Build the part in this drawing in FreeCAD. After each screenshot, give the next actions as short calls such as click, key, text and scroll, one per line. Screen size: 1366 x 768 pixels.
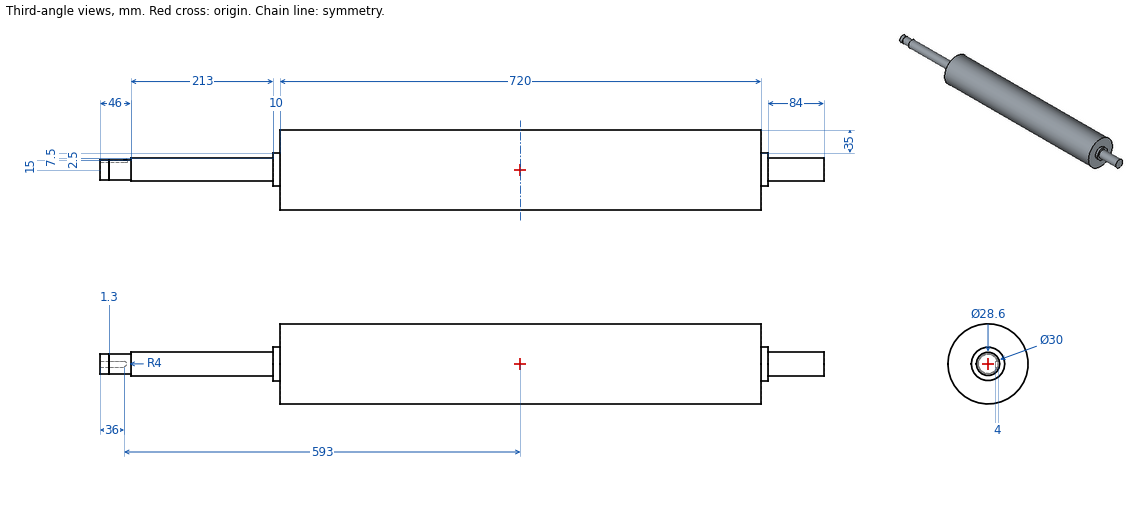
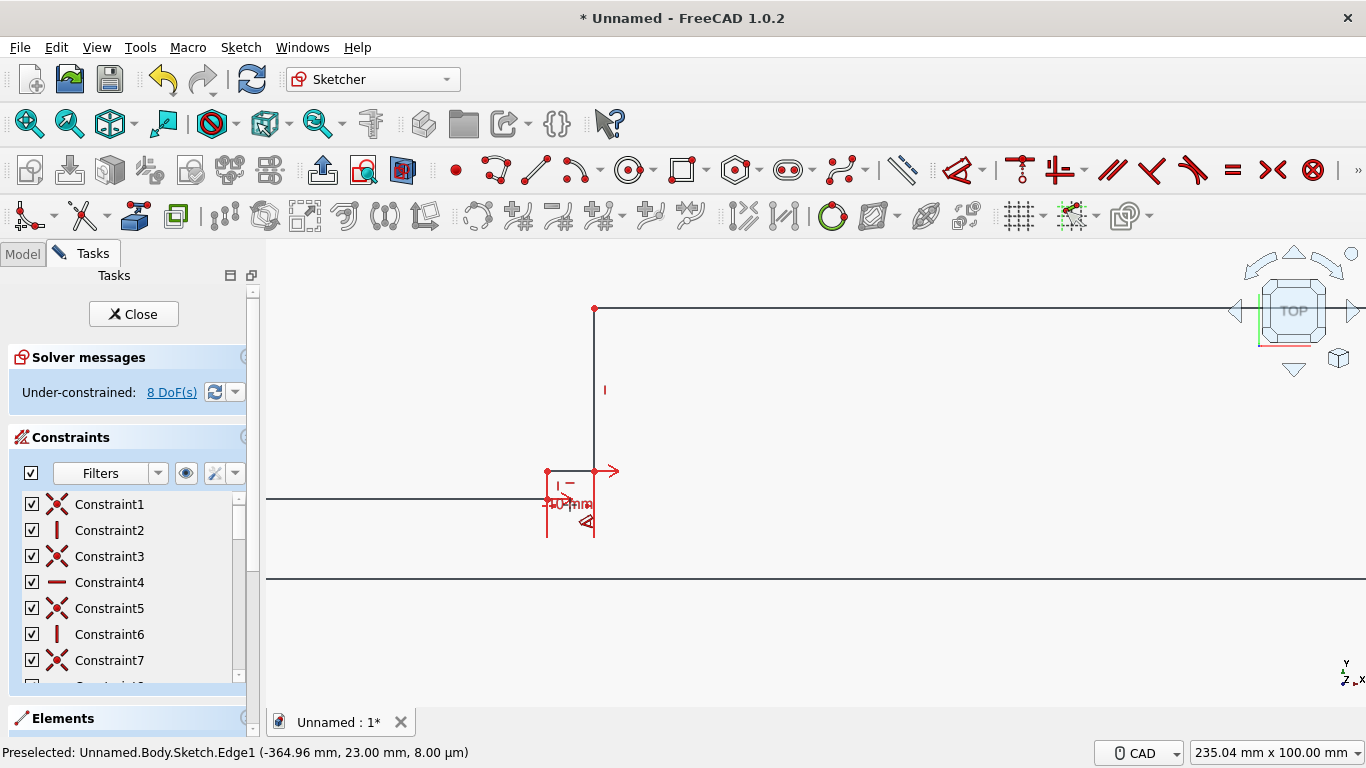
scroll(572, 478, down, 10)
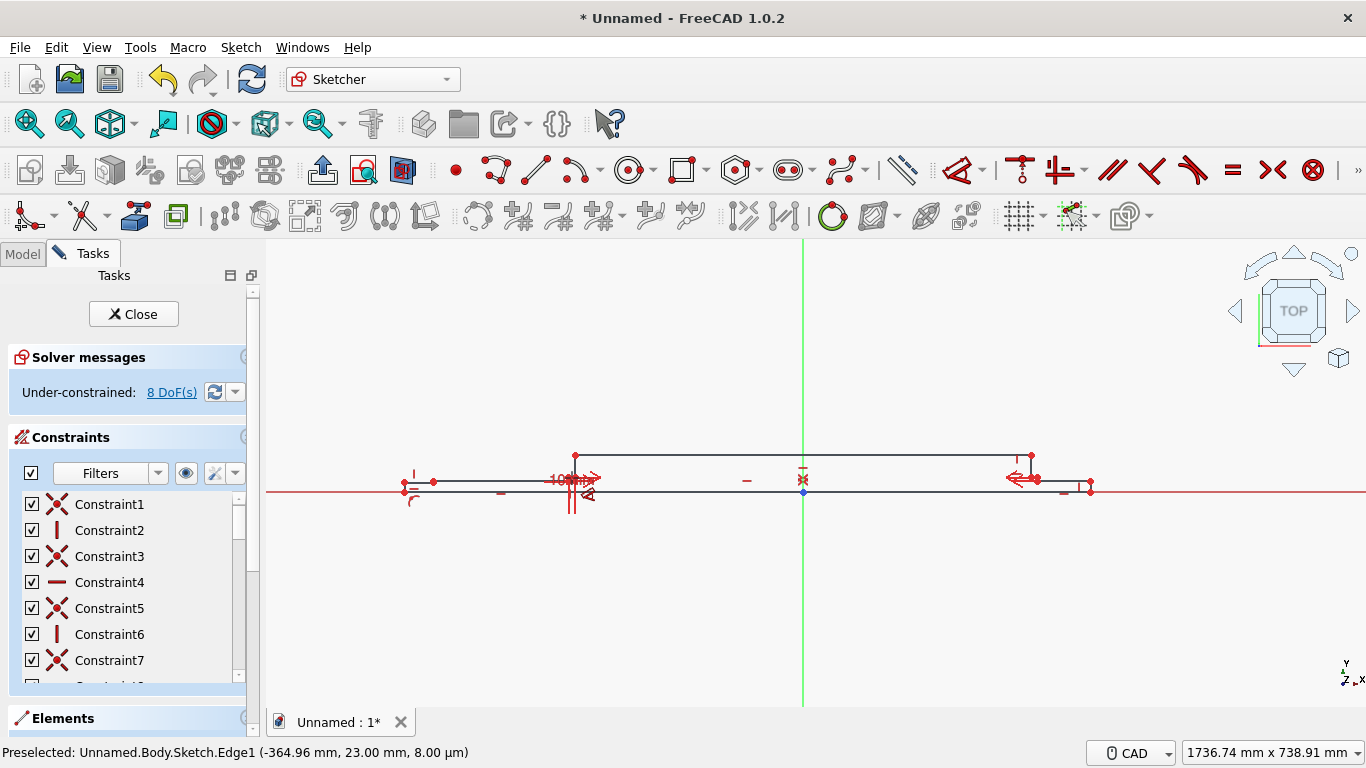
scroll(425, 483, up, 3)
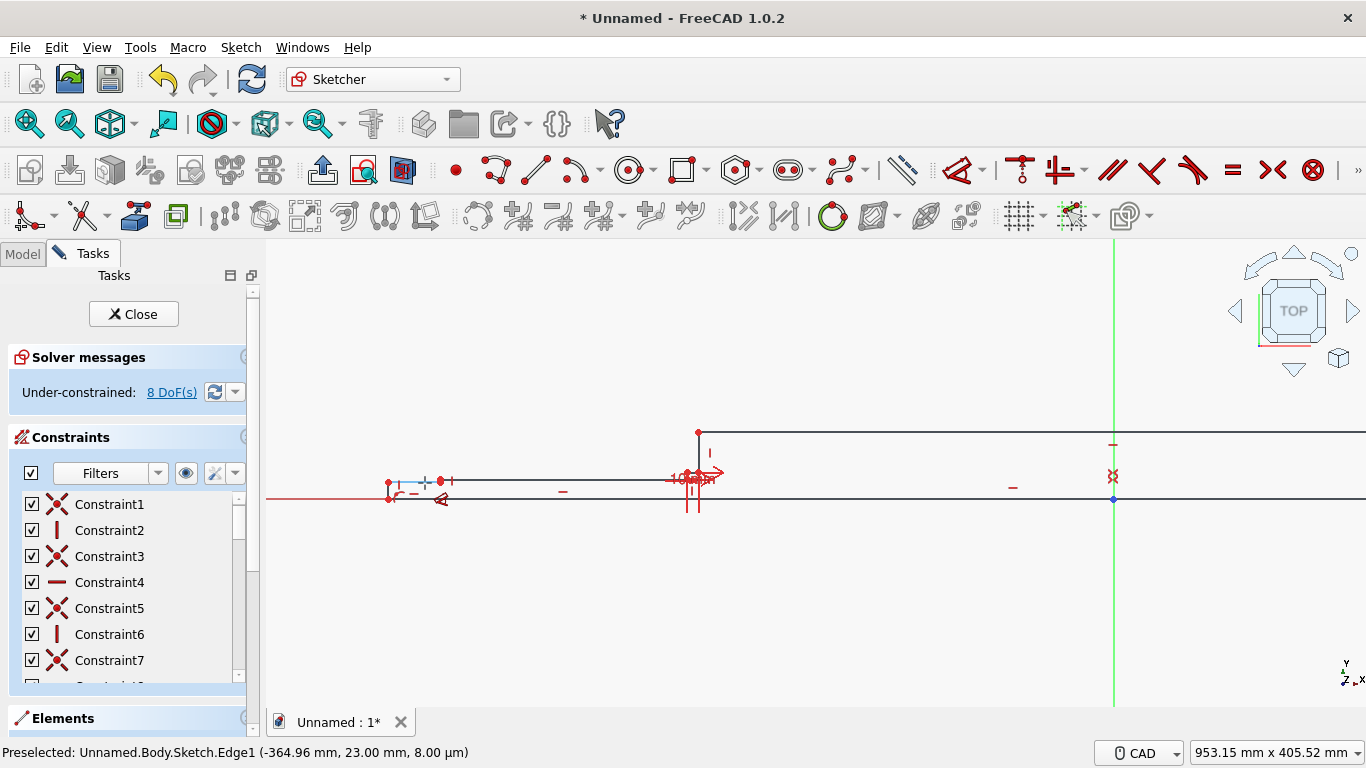
click(425, 482)
click(414, 516)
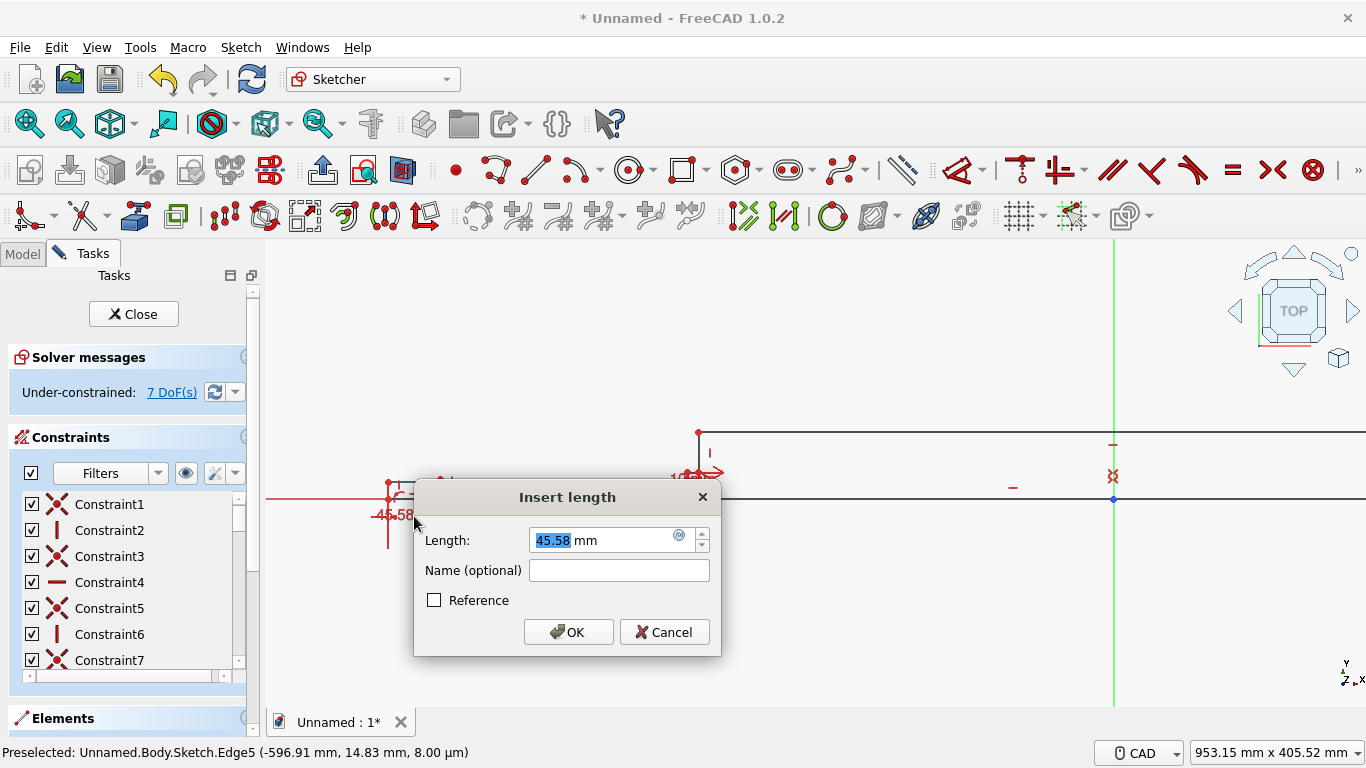
text(46)
key(Return)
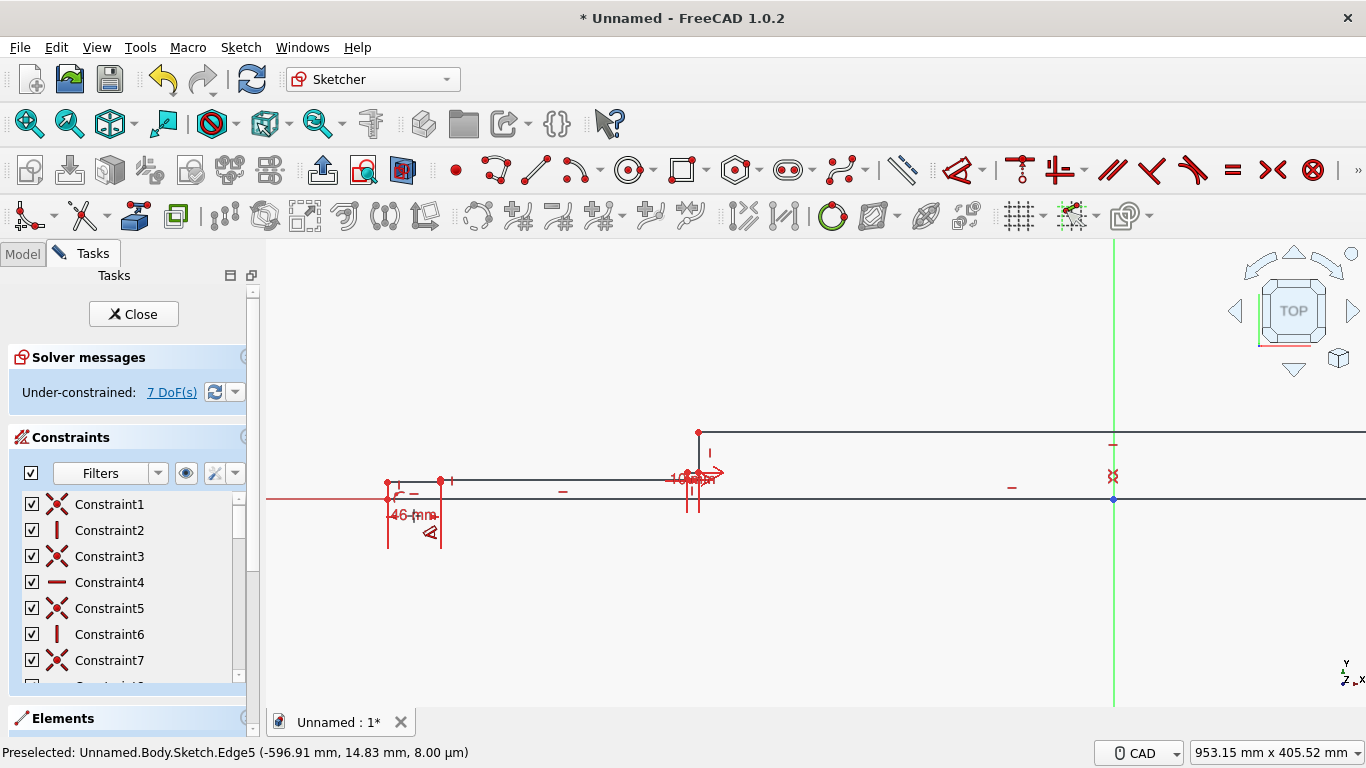
scroll(388, 491, up, 5)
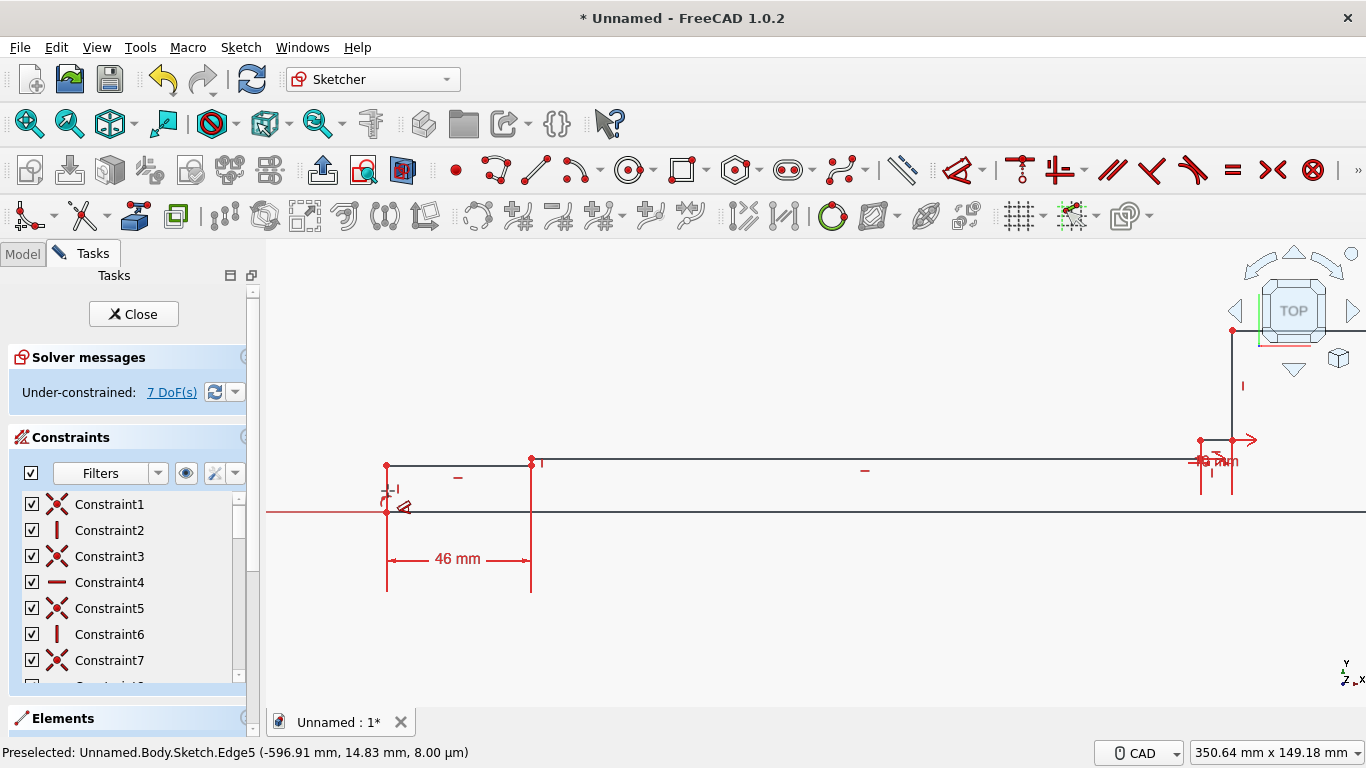
click(387, 489)
click(353, 489)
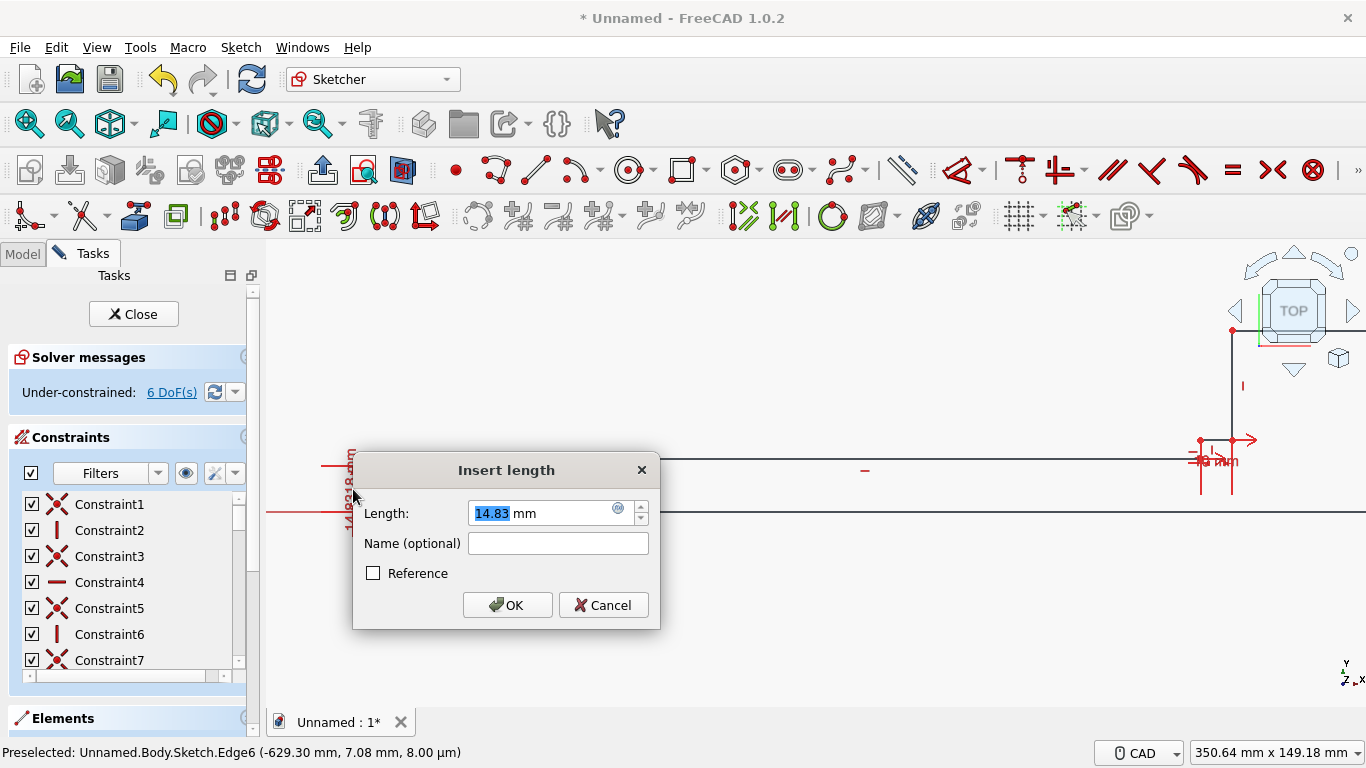
text(15)
key(Return)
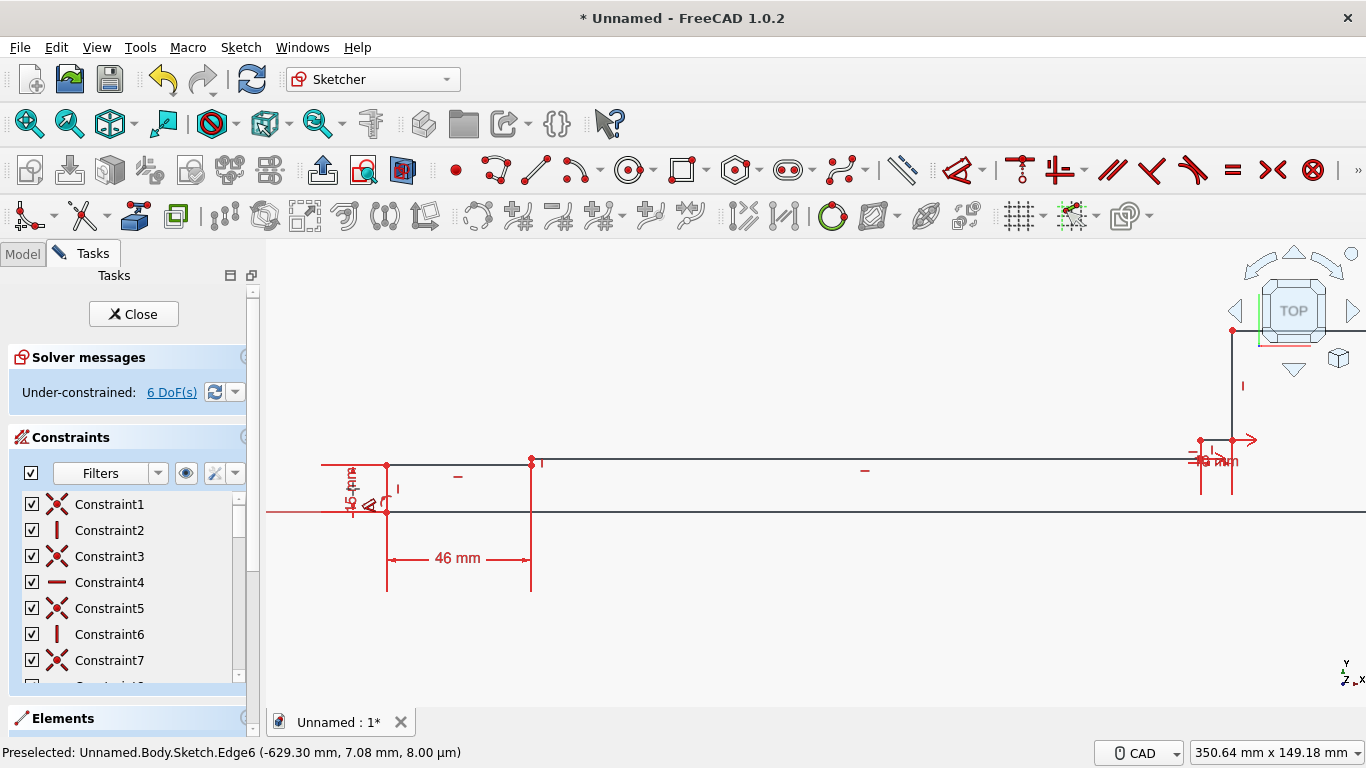
scroll(409, 487, down, 8)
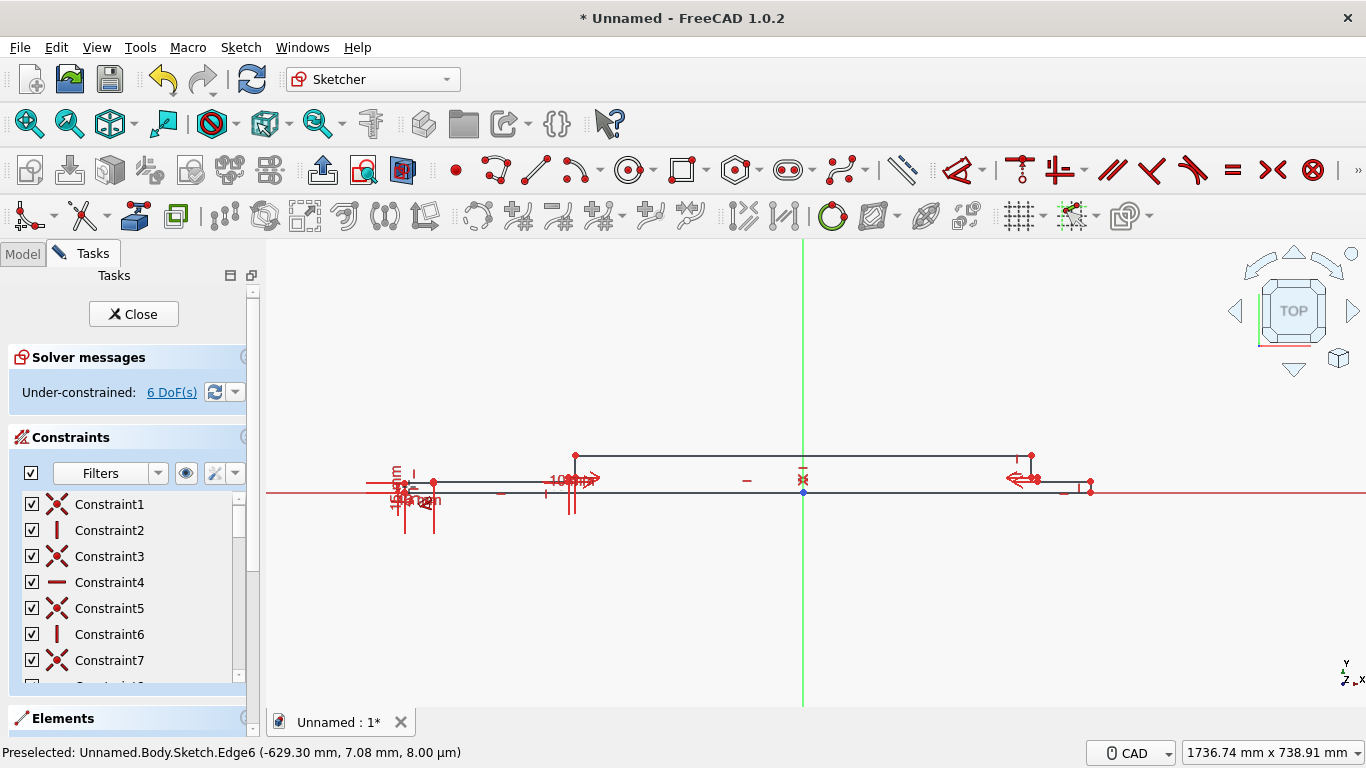
scroll(1075, 482, up, 2)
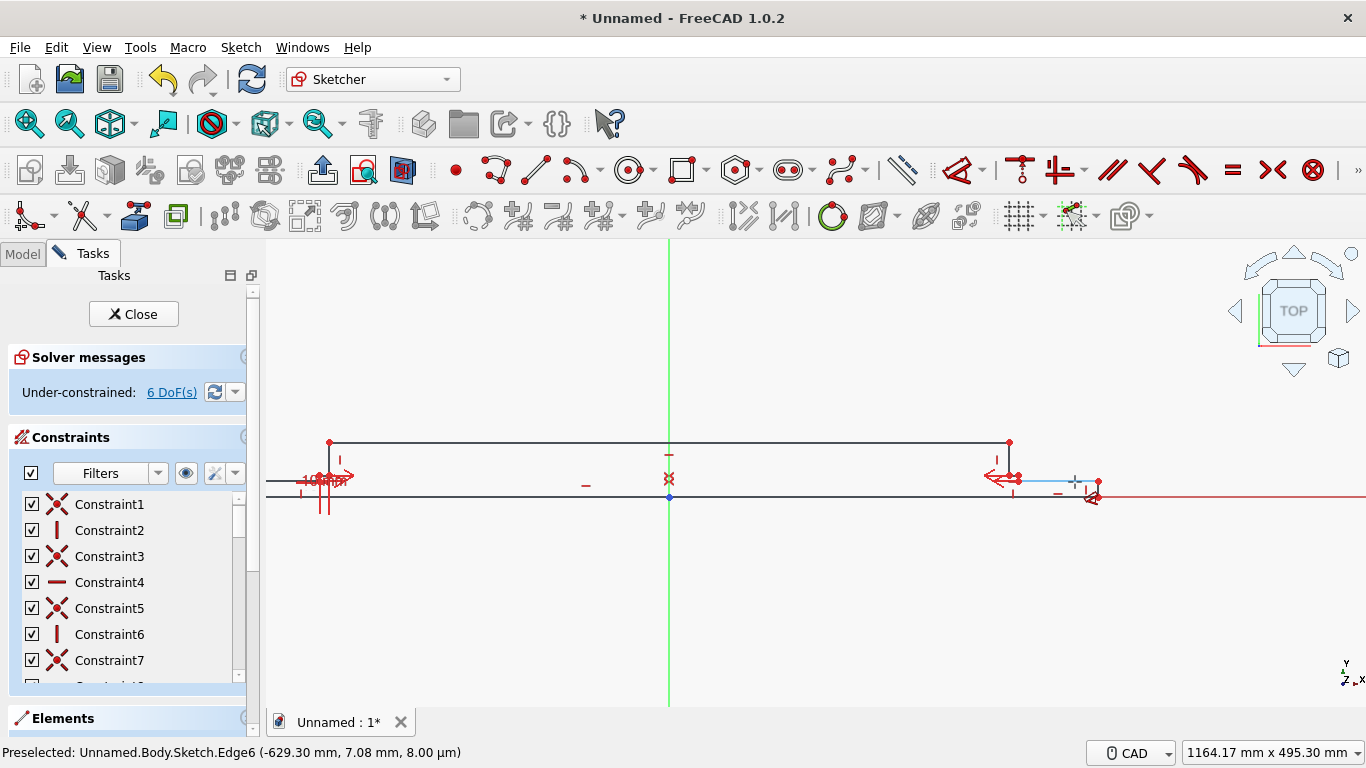
click(1074, 481)
click(1058, 515)